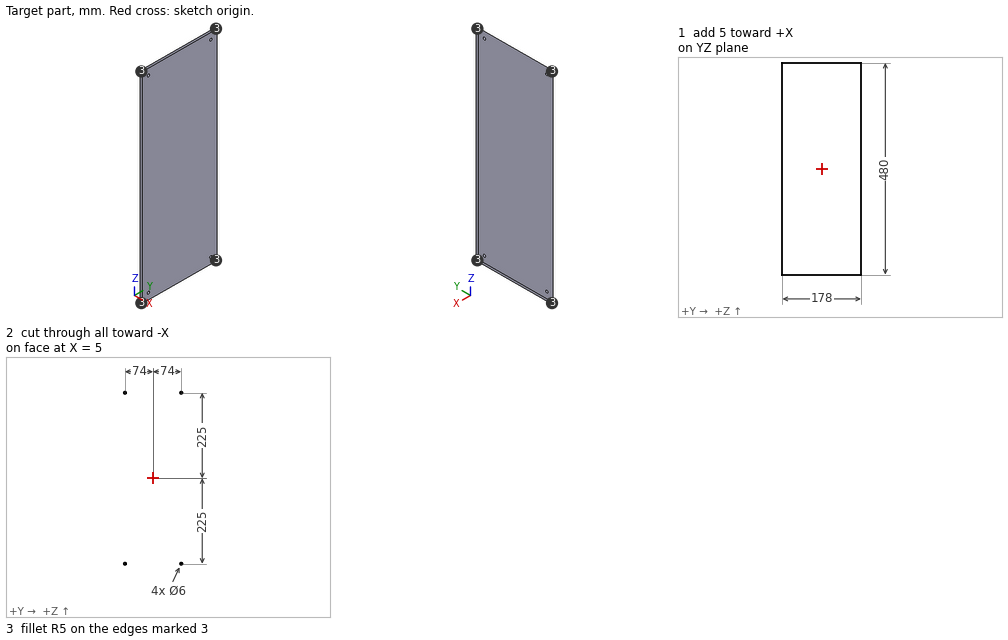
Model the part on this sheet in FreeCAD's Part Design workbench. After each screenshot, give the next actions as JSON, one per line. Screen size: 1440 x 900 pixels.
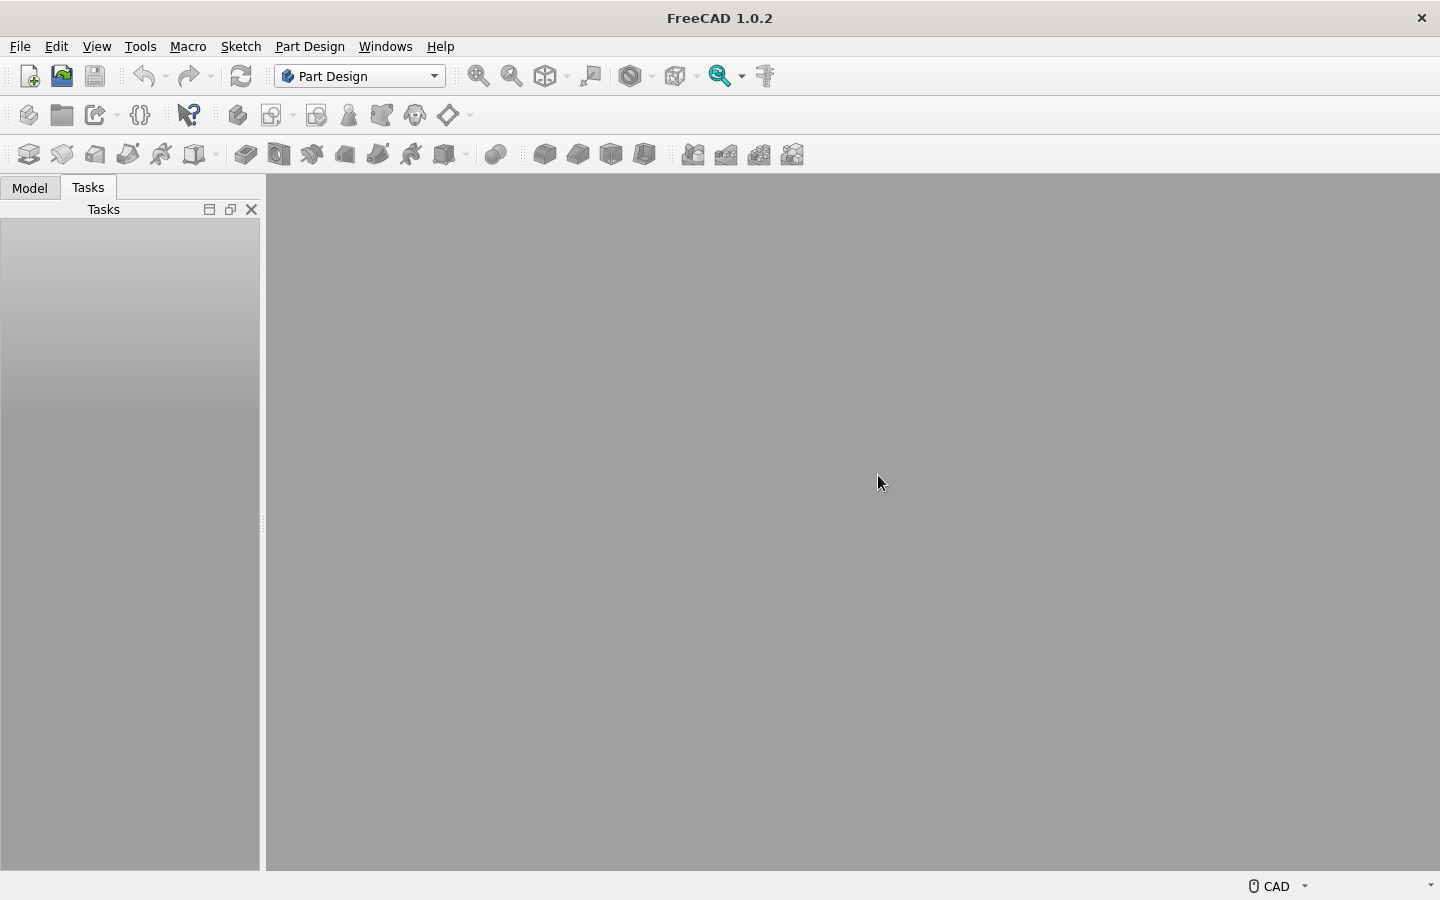
{"action": "left_click", "coordinate": [29, 76]}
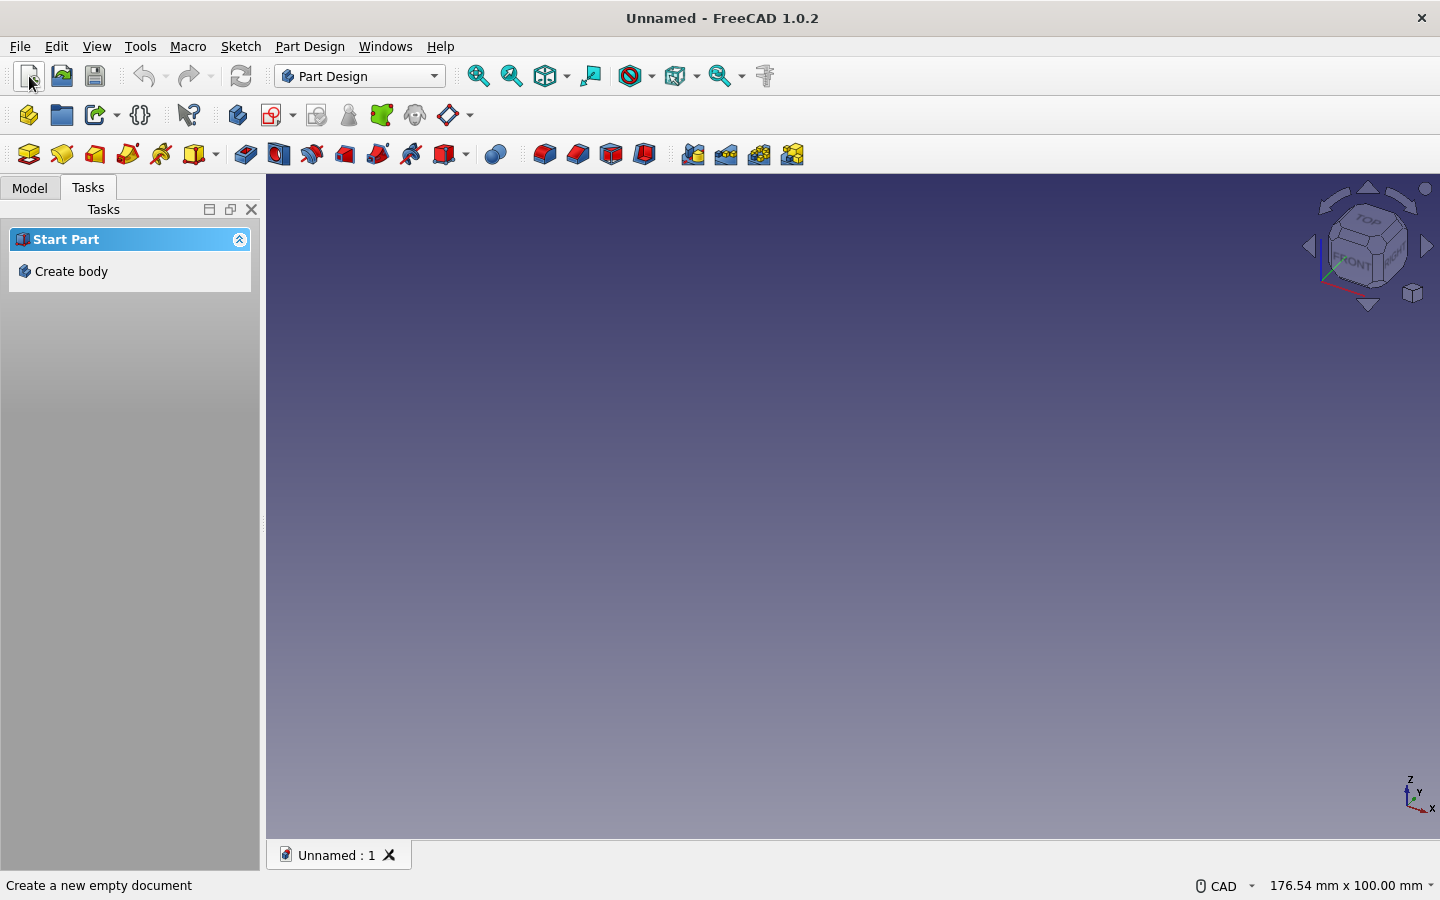
{"action": "left_click", "coordinate": [270, 116]}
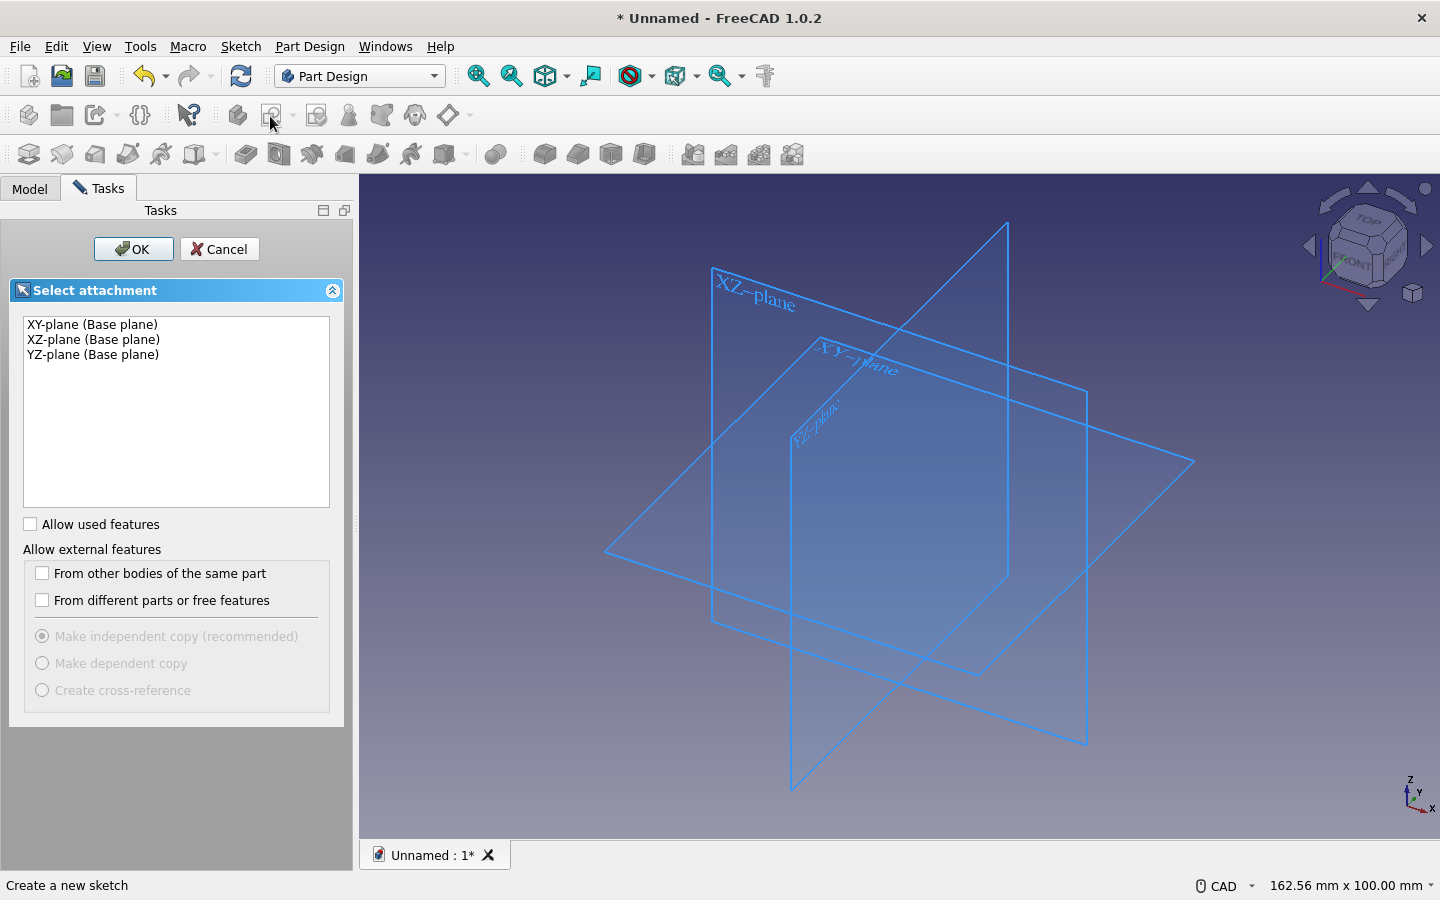
{"action": "left_click", "coordinate": [84, 354]}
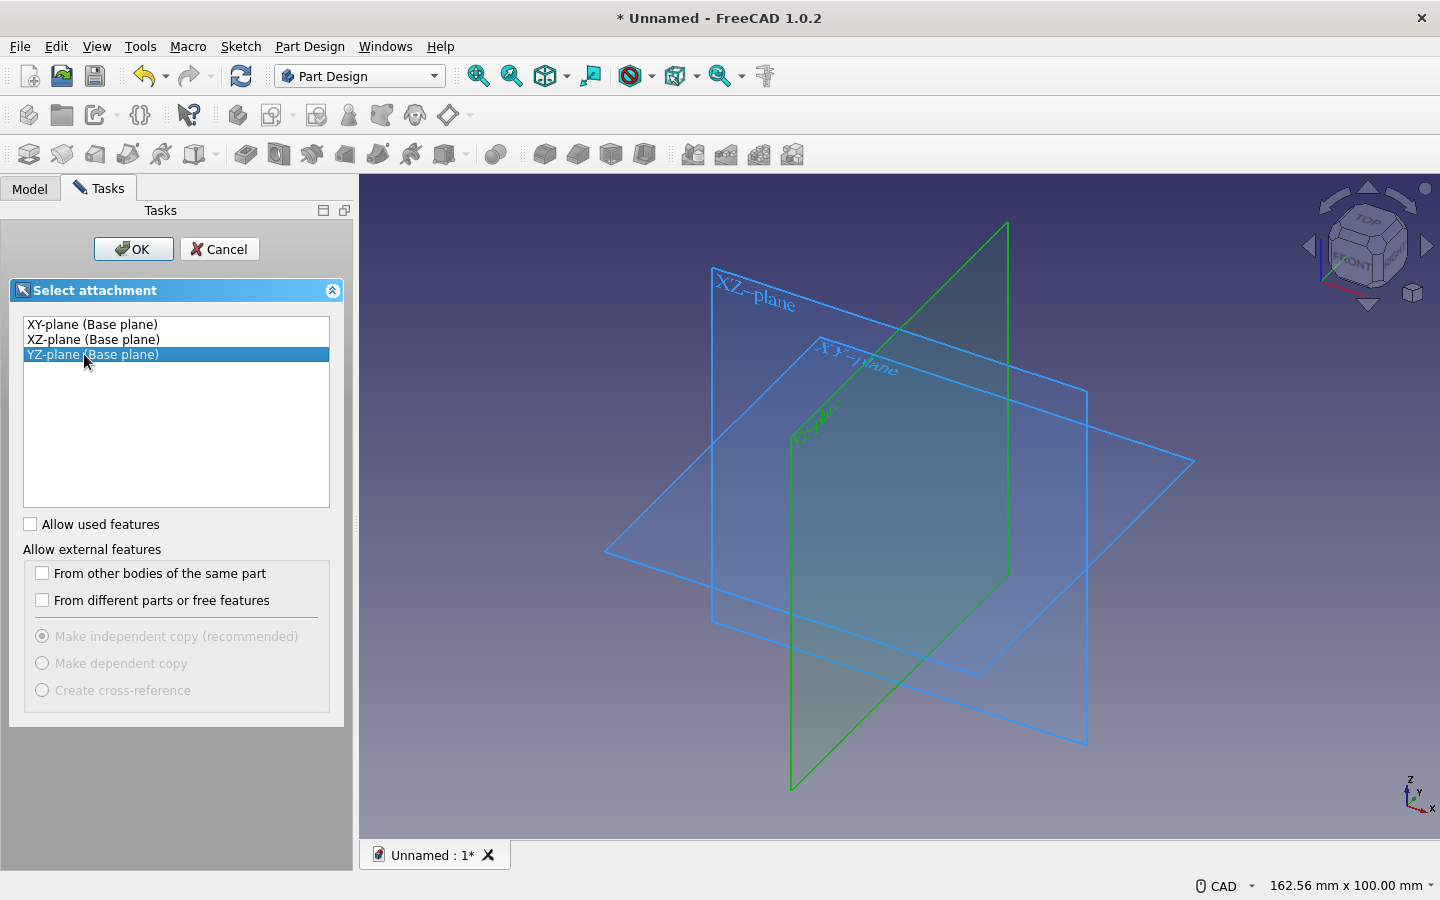
{"action": "left_click", "coordinate": [134, 249]}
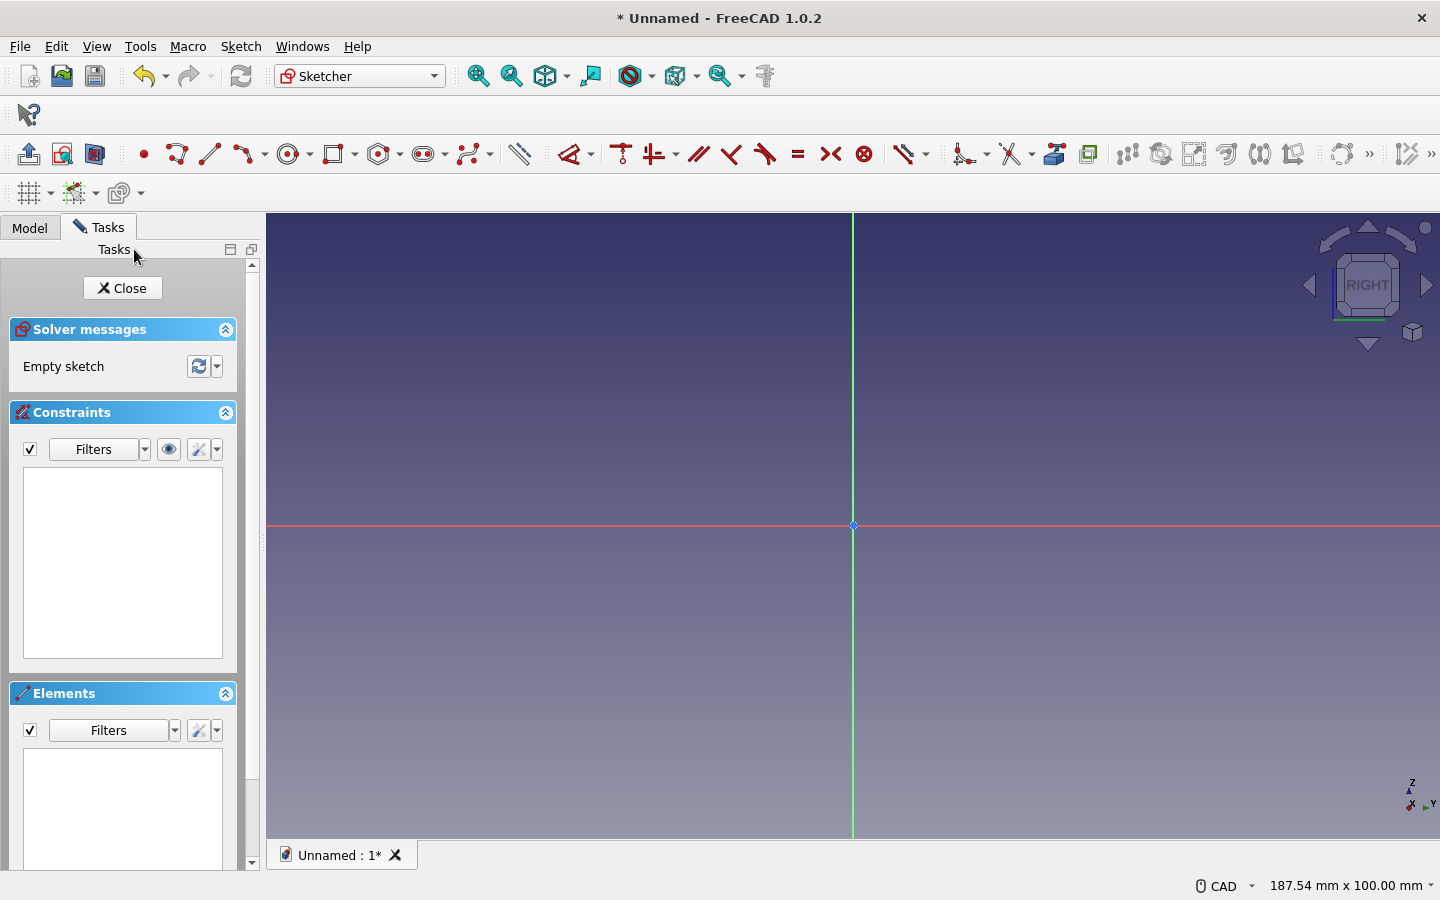
{"action": "scroll", "coordinate": [774, 526], "scroll_direction": "down", "scroll_amount": 10}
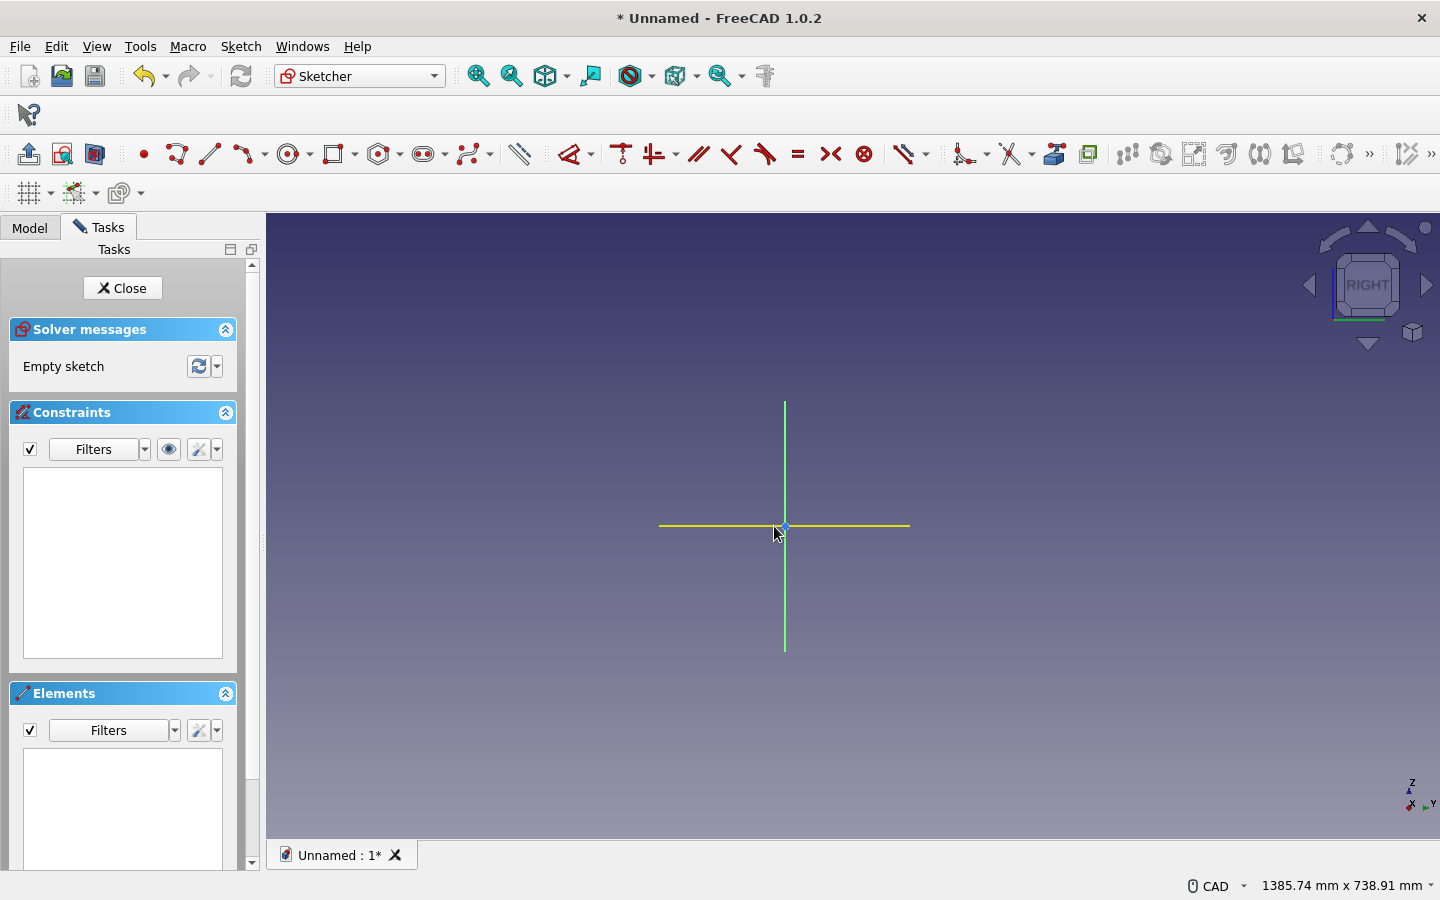
{"action": "left_click", "coordinate": [354, 154]}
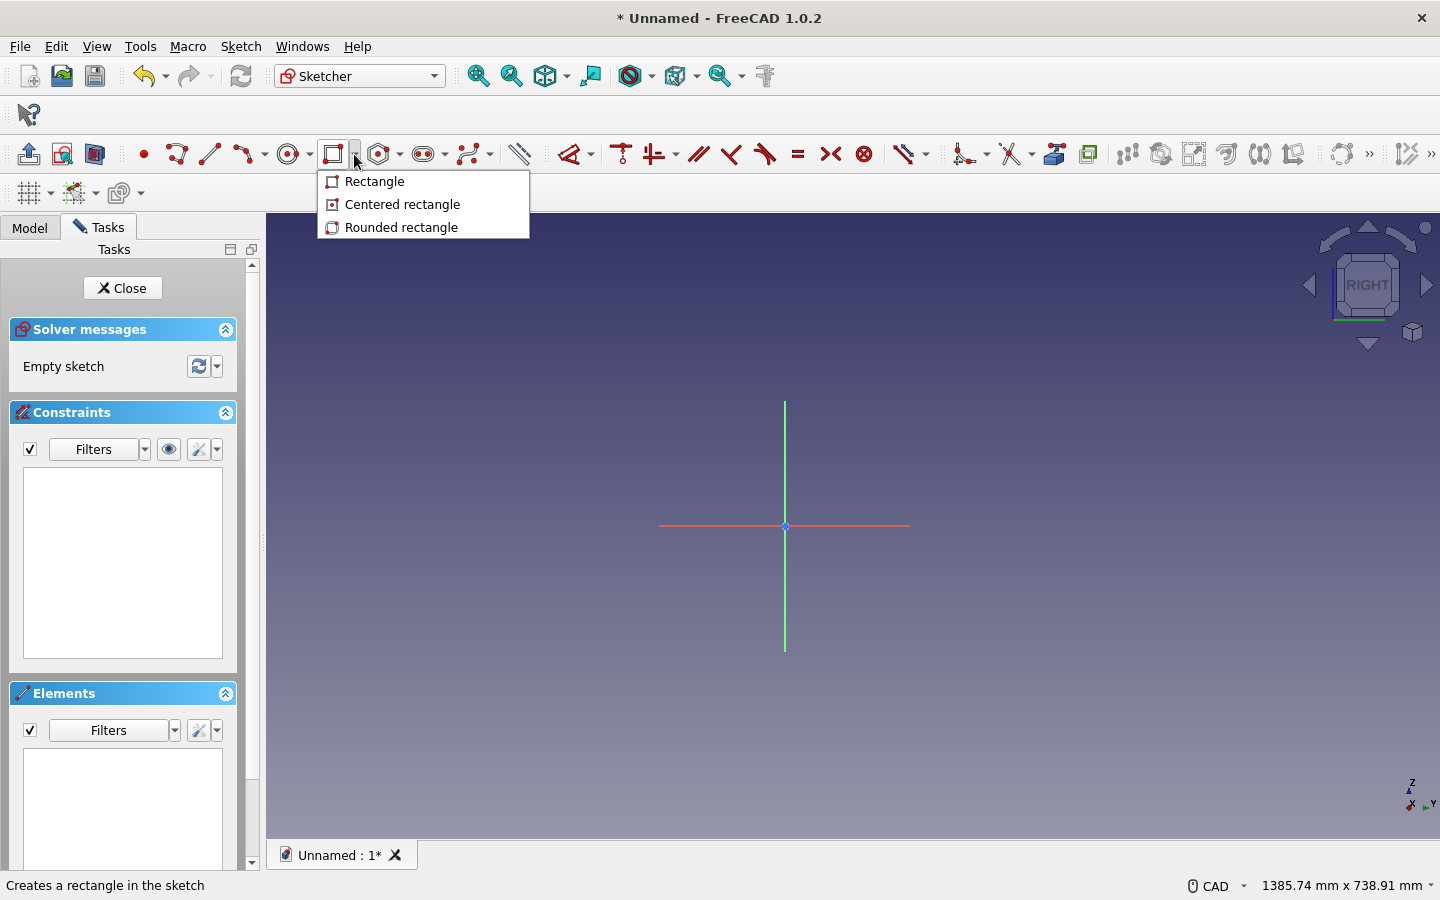
{"action": "left_click", "coordinate": [424, 204]}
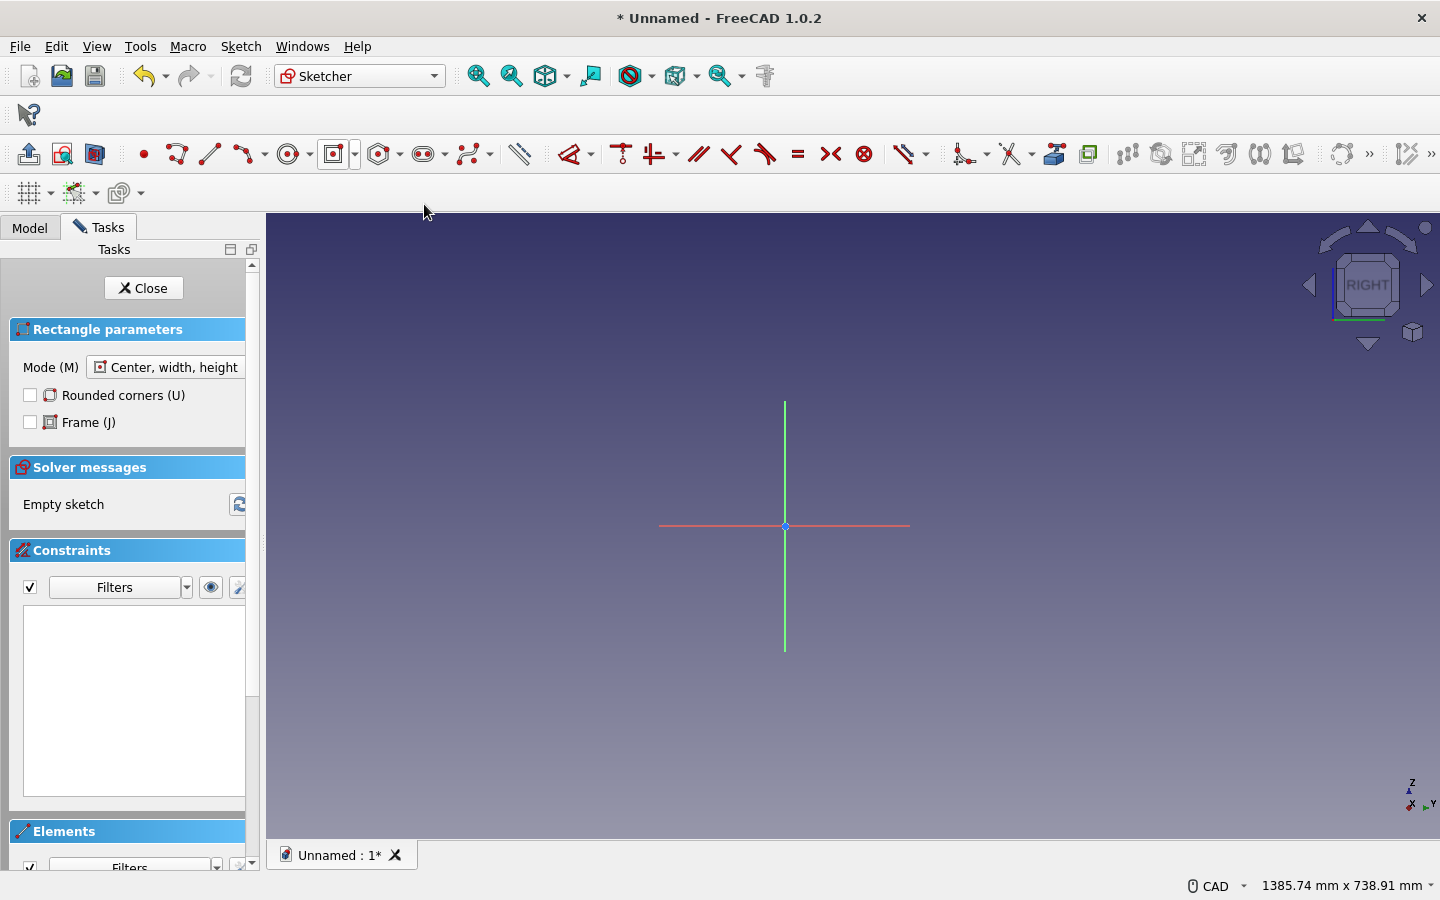
{"action": "left_click", "coordinate": [785, 526]}
{"action": "left_click", "coordinate": [860, 323]}
{"action": "key", "text": "Escape"}